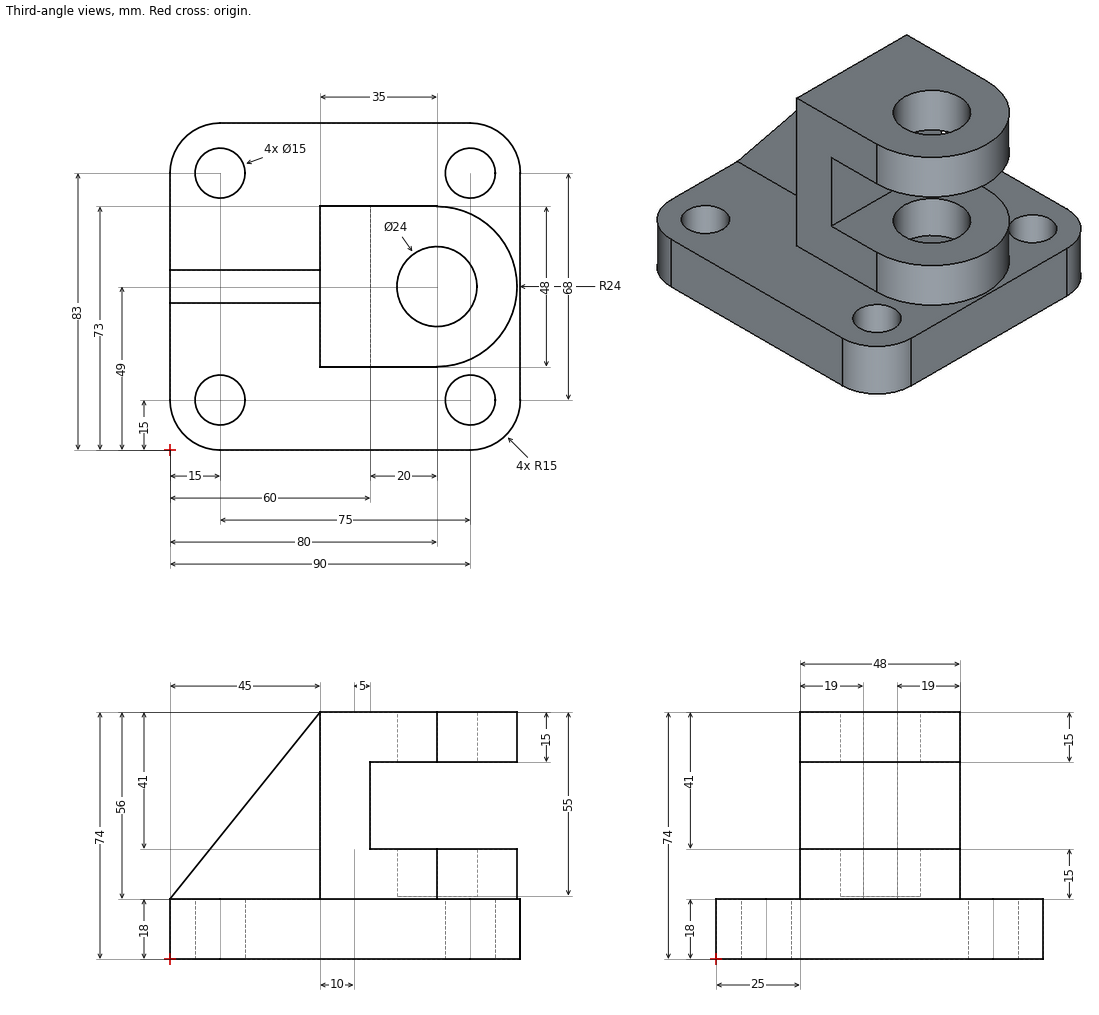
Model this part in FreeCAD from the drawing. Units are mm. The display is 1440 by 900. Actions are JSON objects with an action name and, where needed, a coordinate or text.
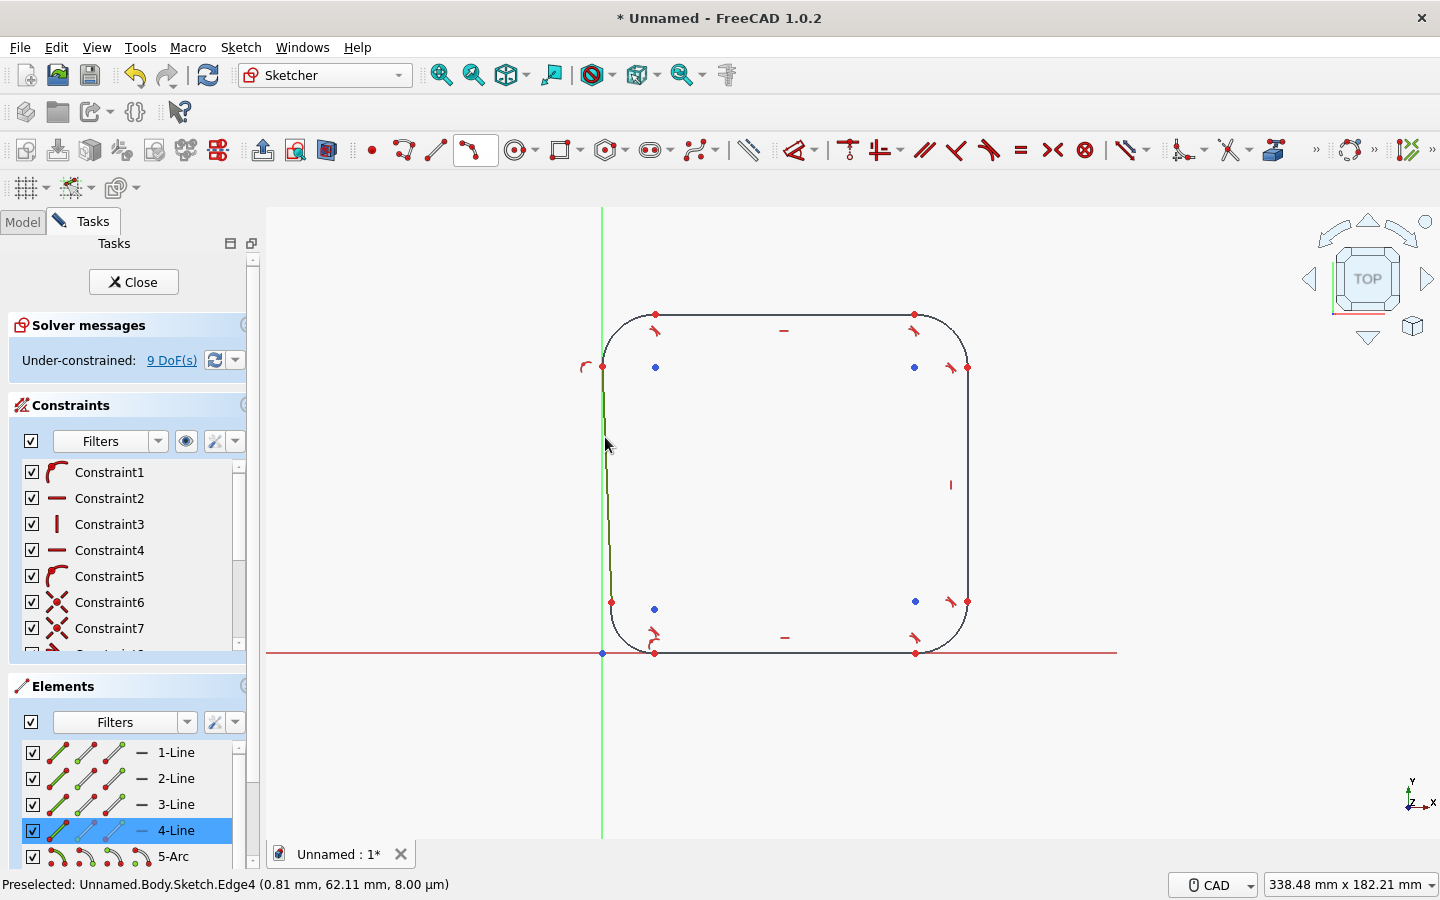
{"action": "left_click", "coordinate": [631, 320]}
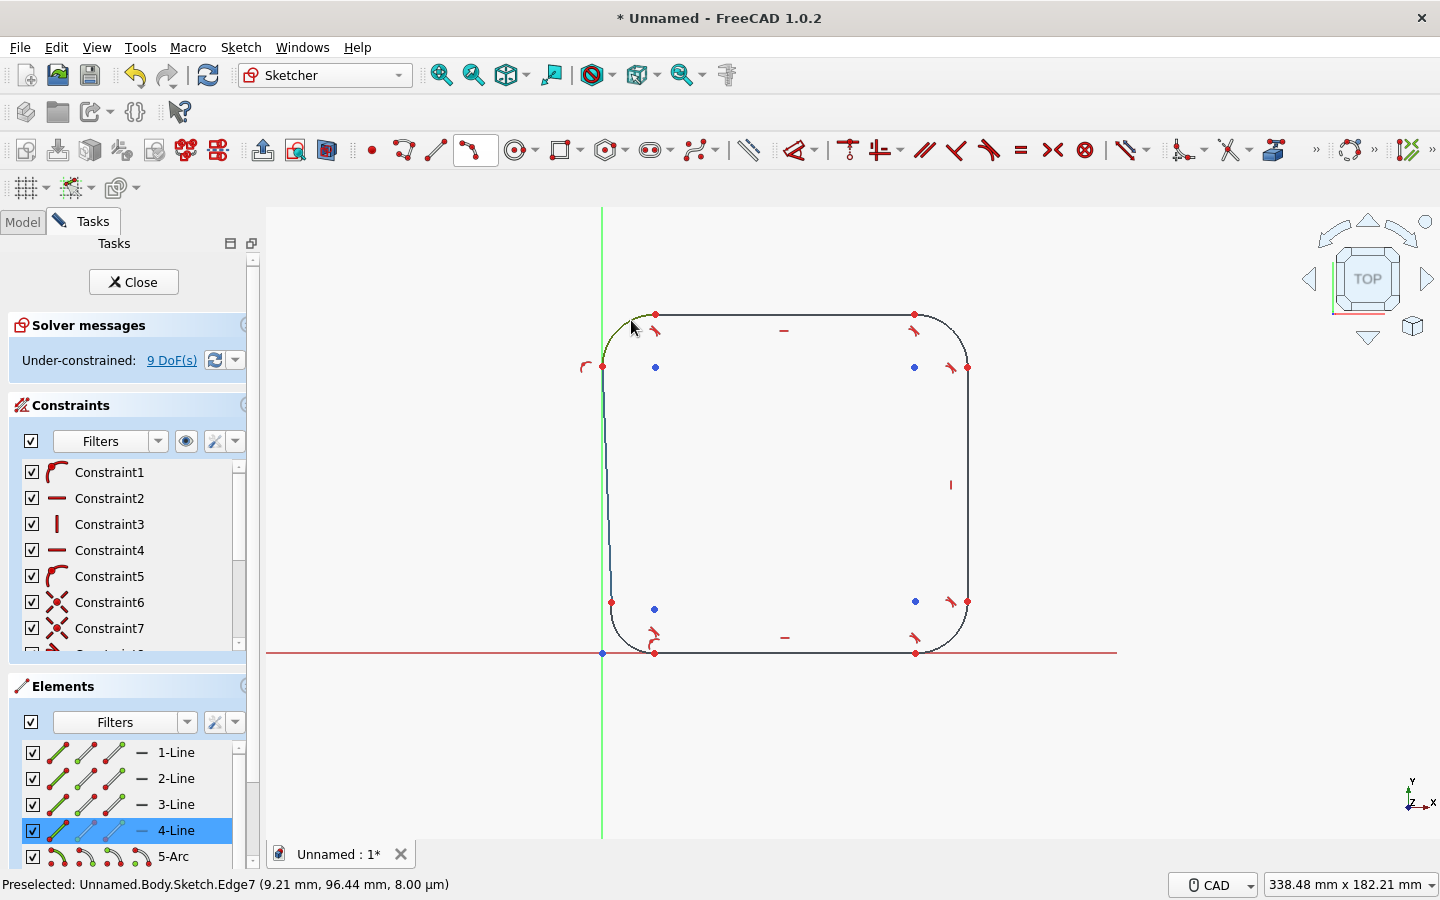
{"action": "left_click", "coordinate": [990, 150]}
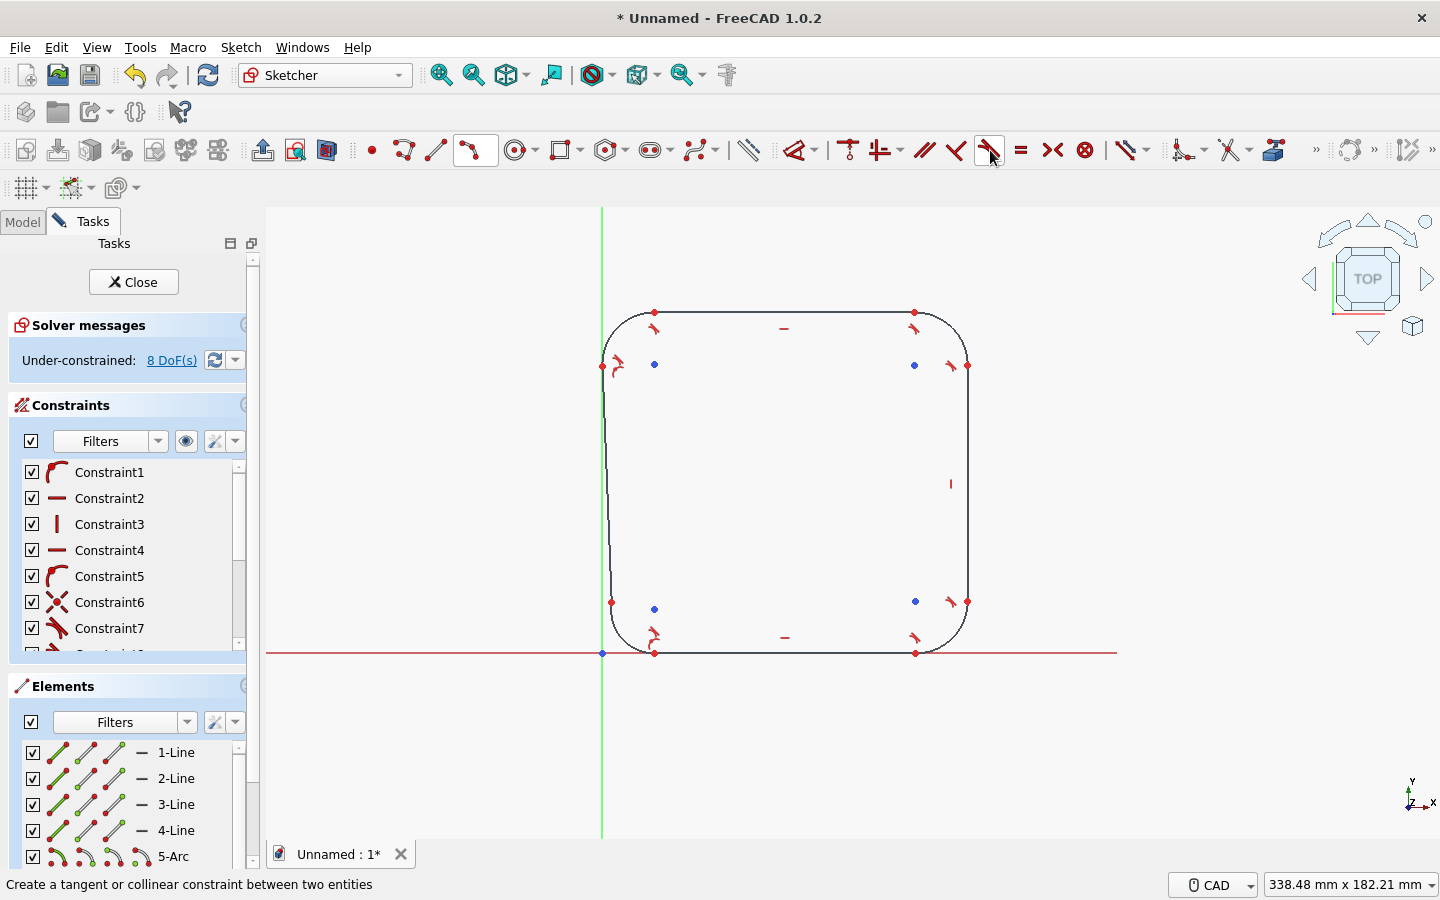
{"action": "left_click", "coordinate": [605, 437]}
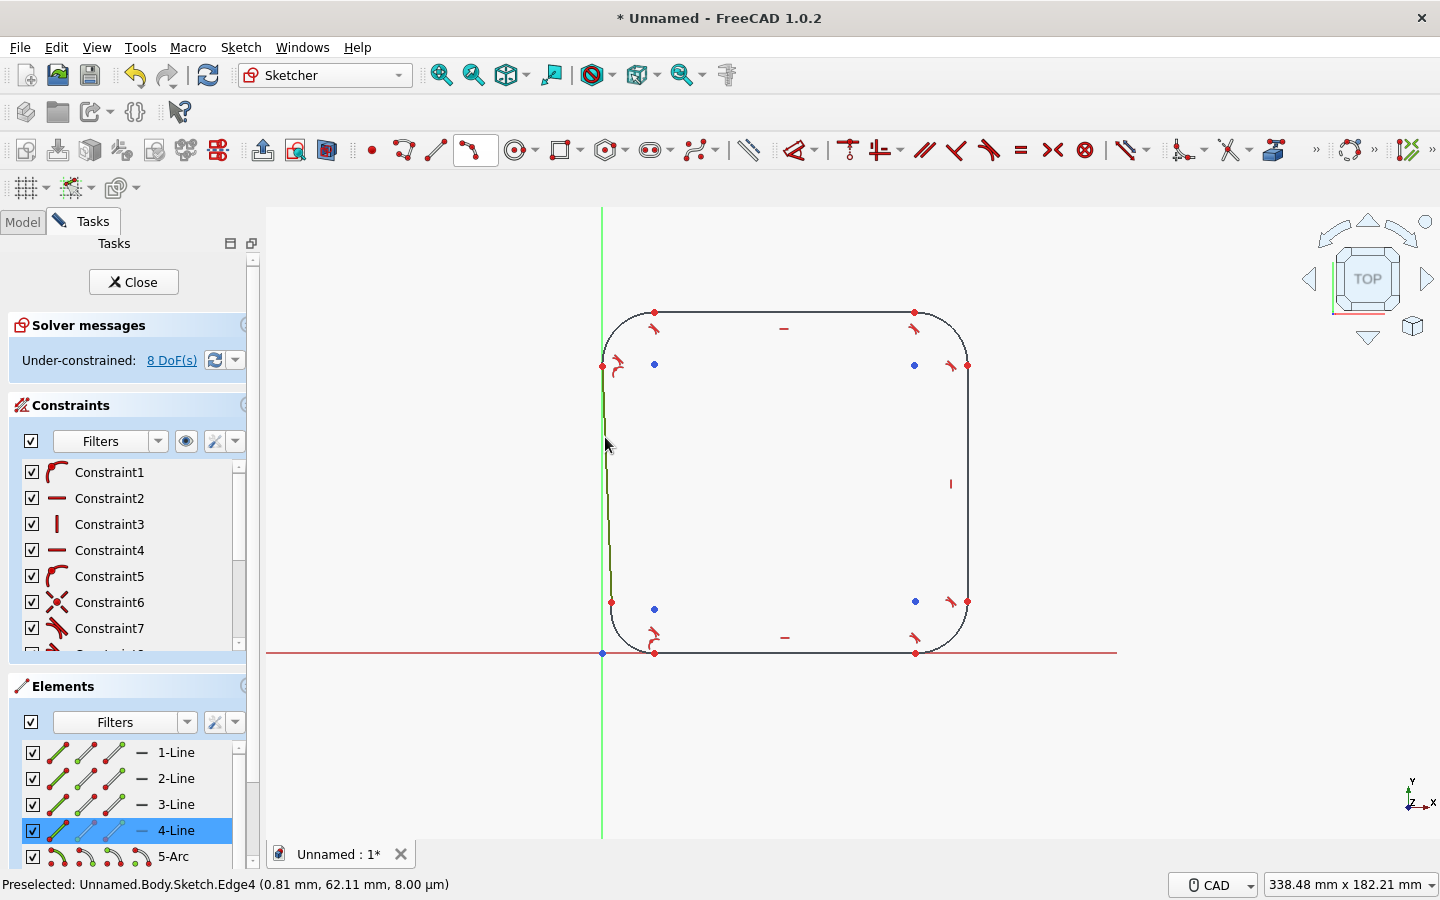
{"action": "left_click", "coordinate": [614, 625]}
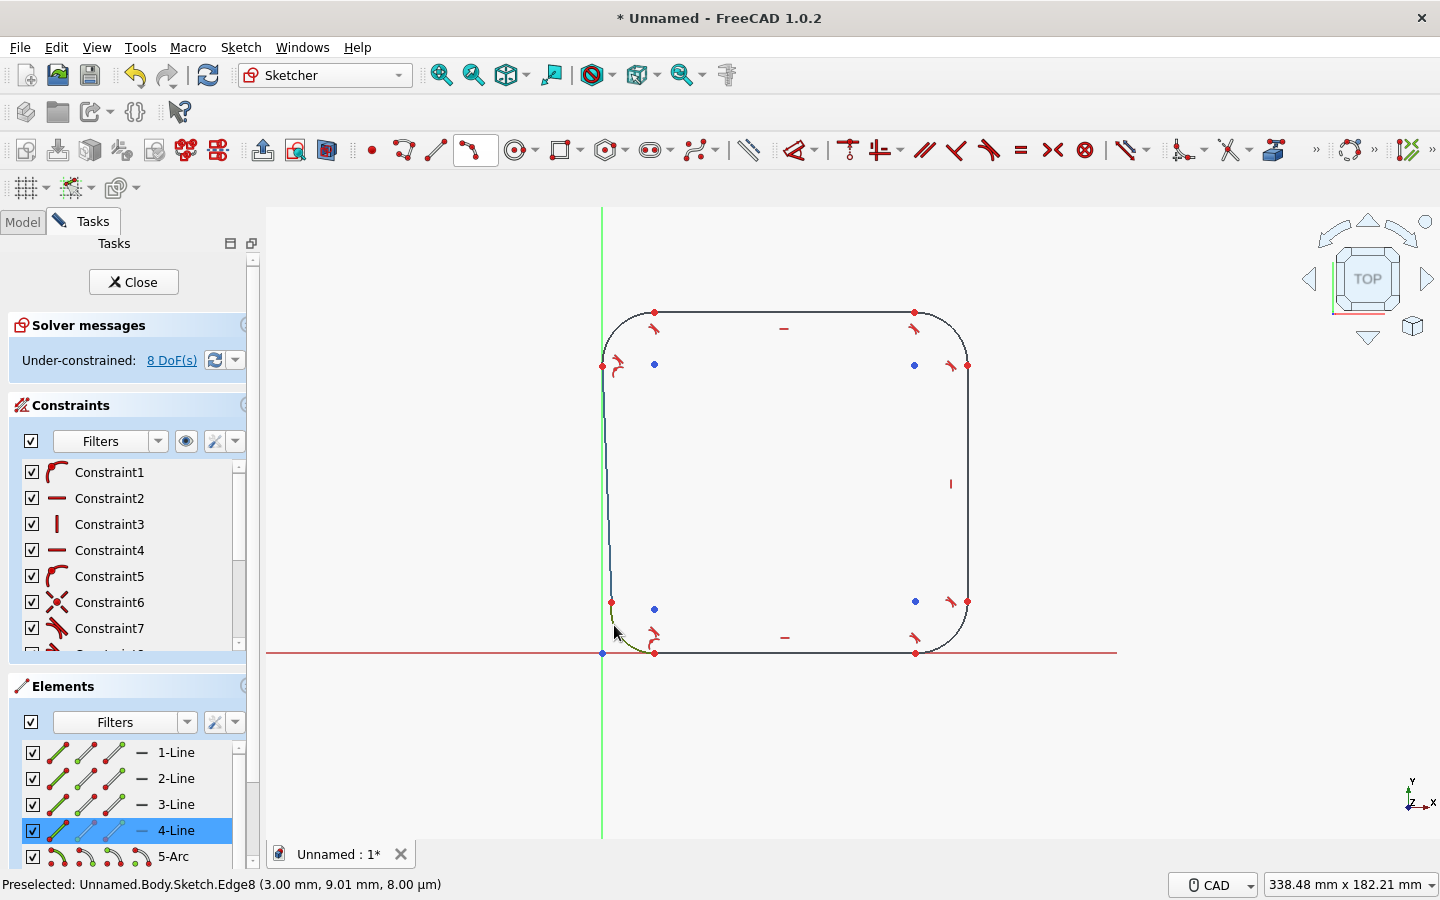
{"action": "left_click", "coordinate": [990, 150]}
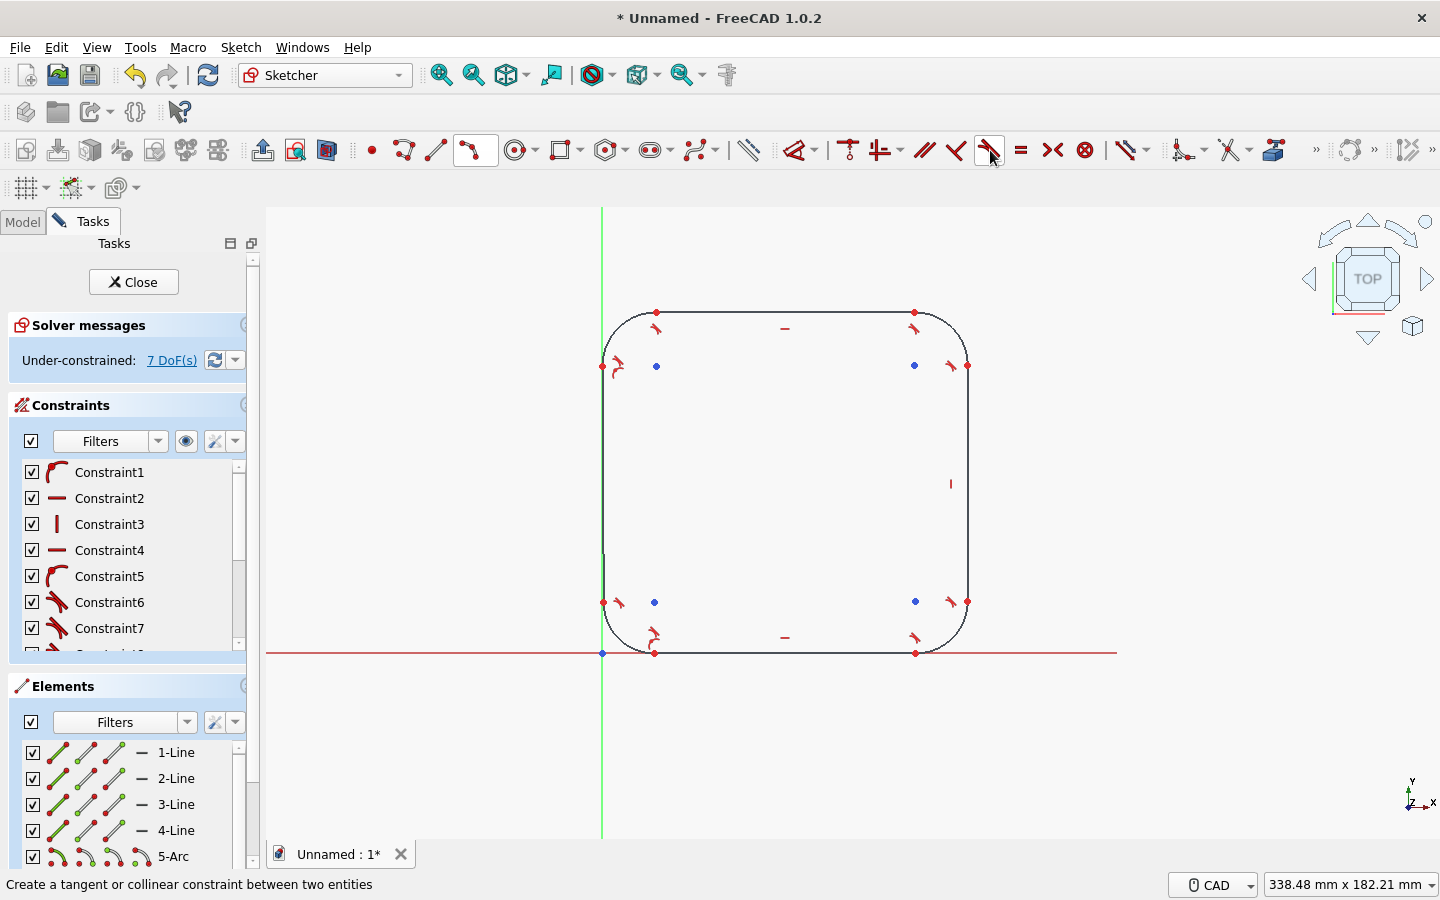
{"action": "left_click", "coordinate": [603, 437]}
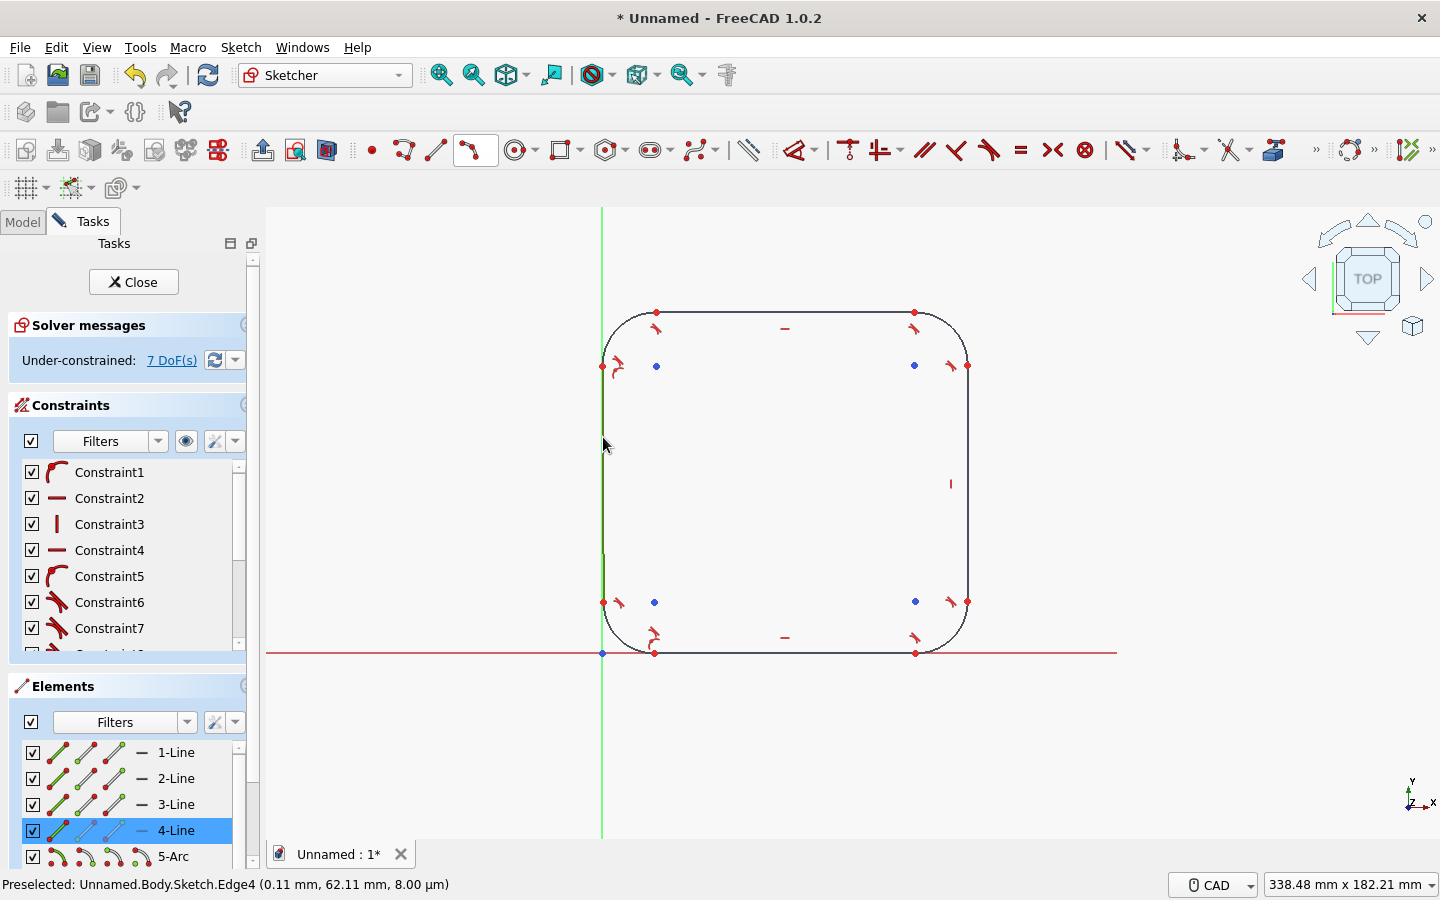
{"action": "left_click", "coordinate": [902, 150]}